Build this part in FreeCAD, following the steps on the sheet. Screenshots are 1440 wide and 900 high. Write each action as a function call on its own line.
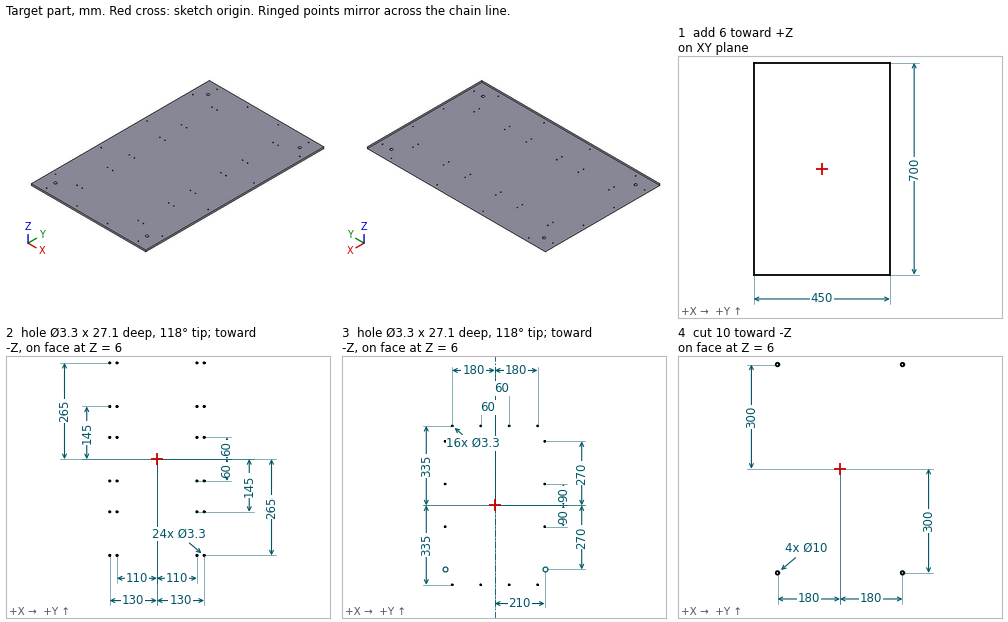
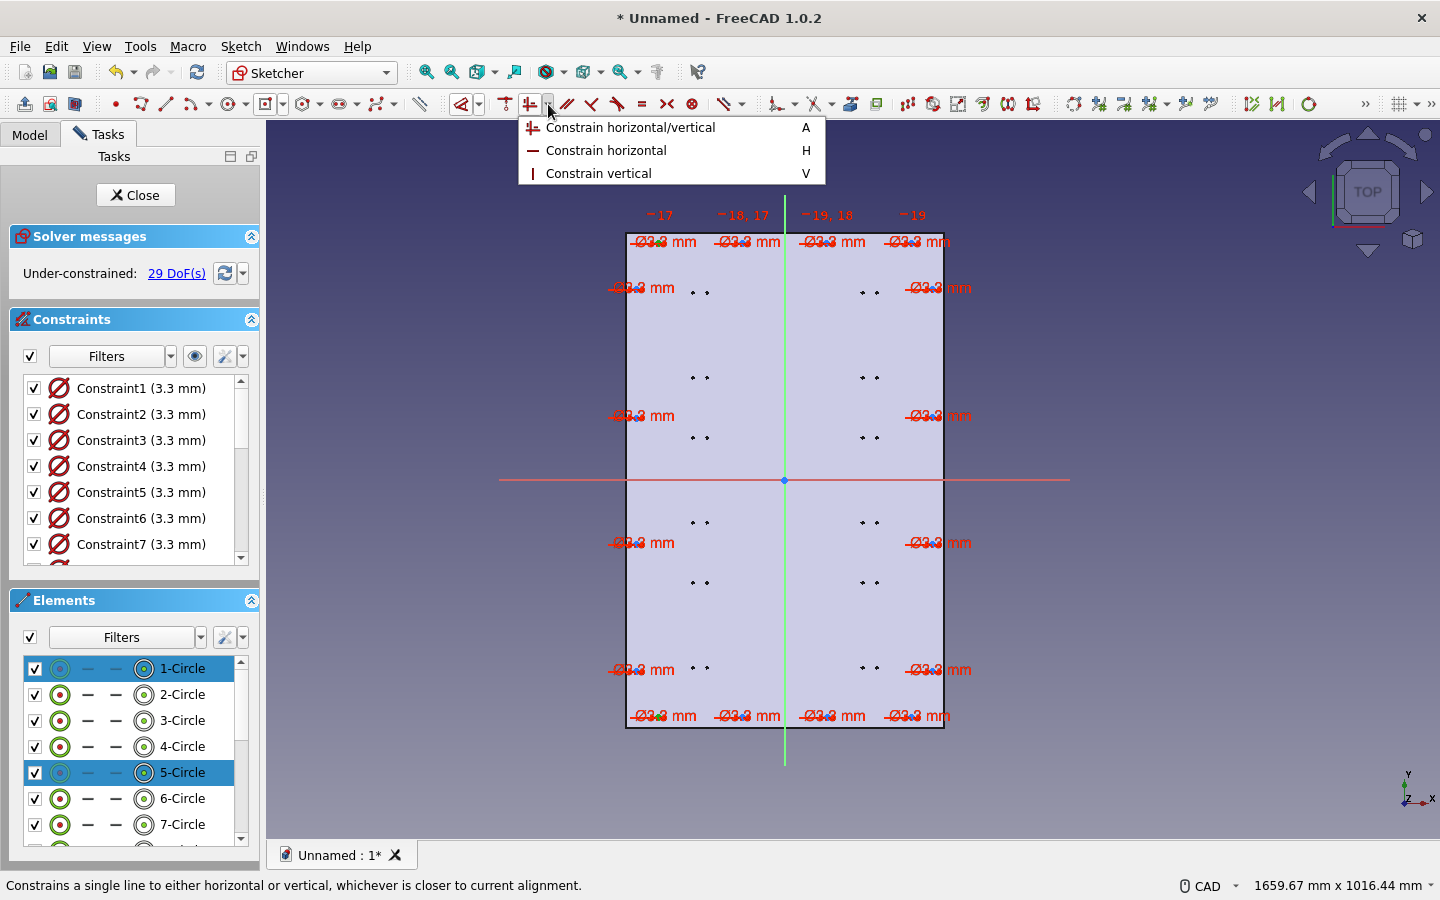
click(672, 174)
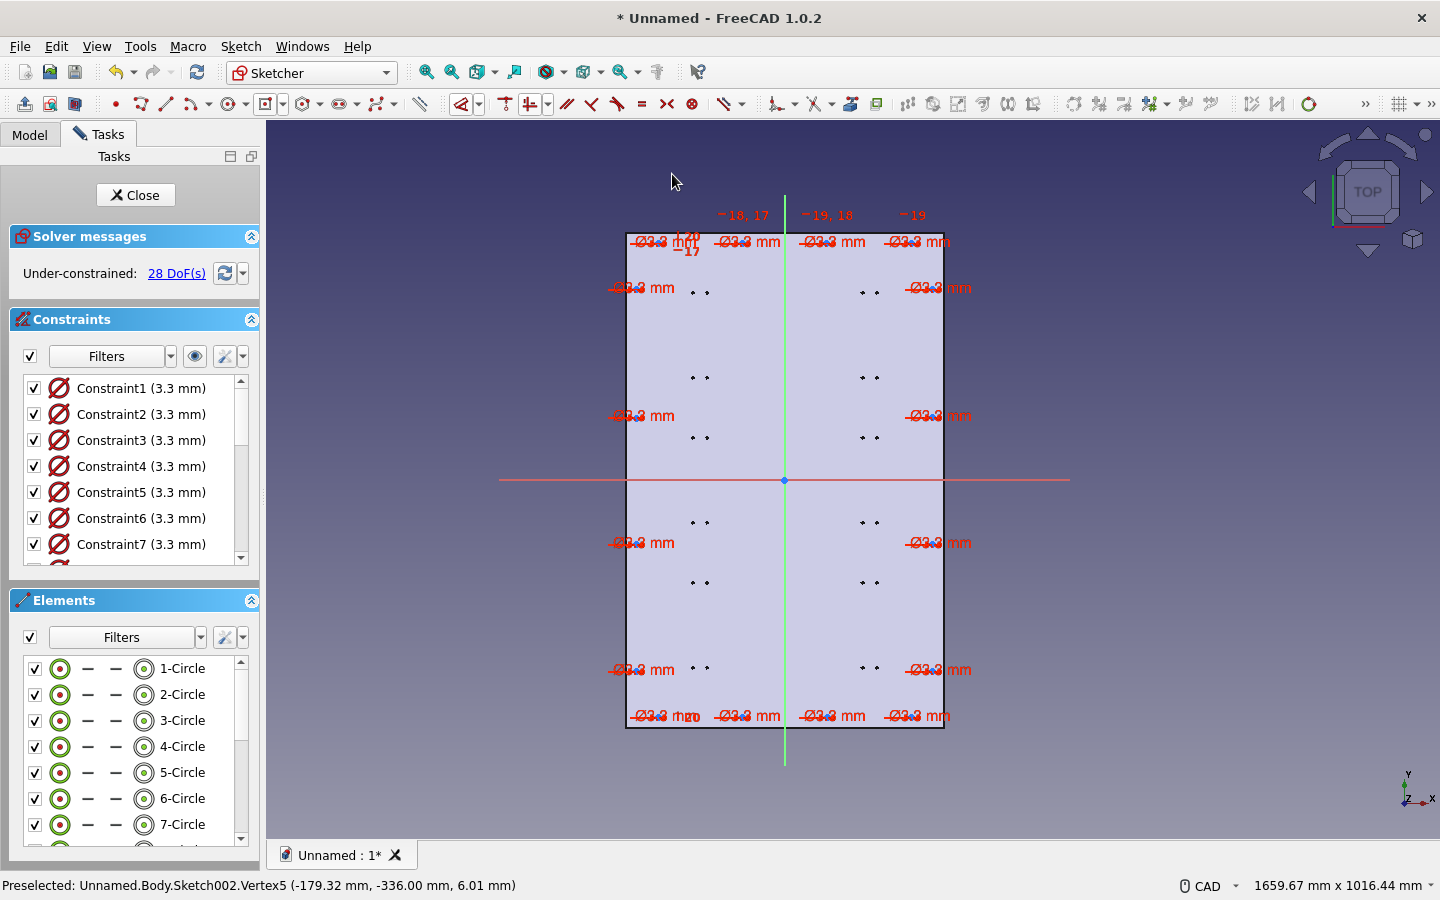
click(742, 244)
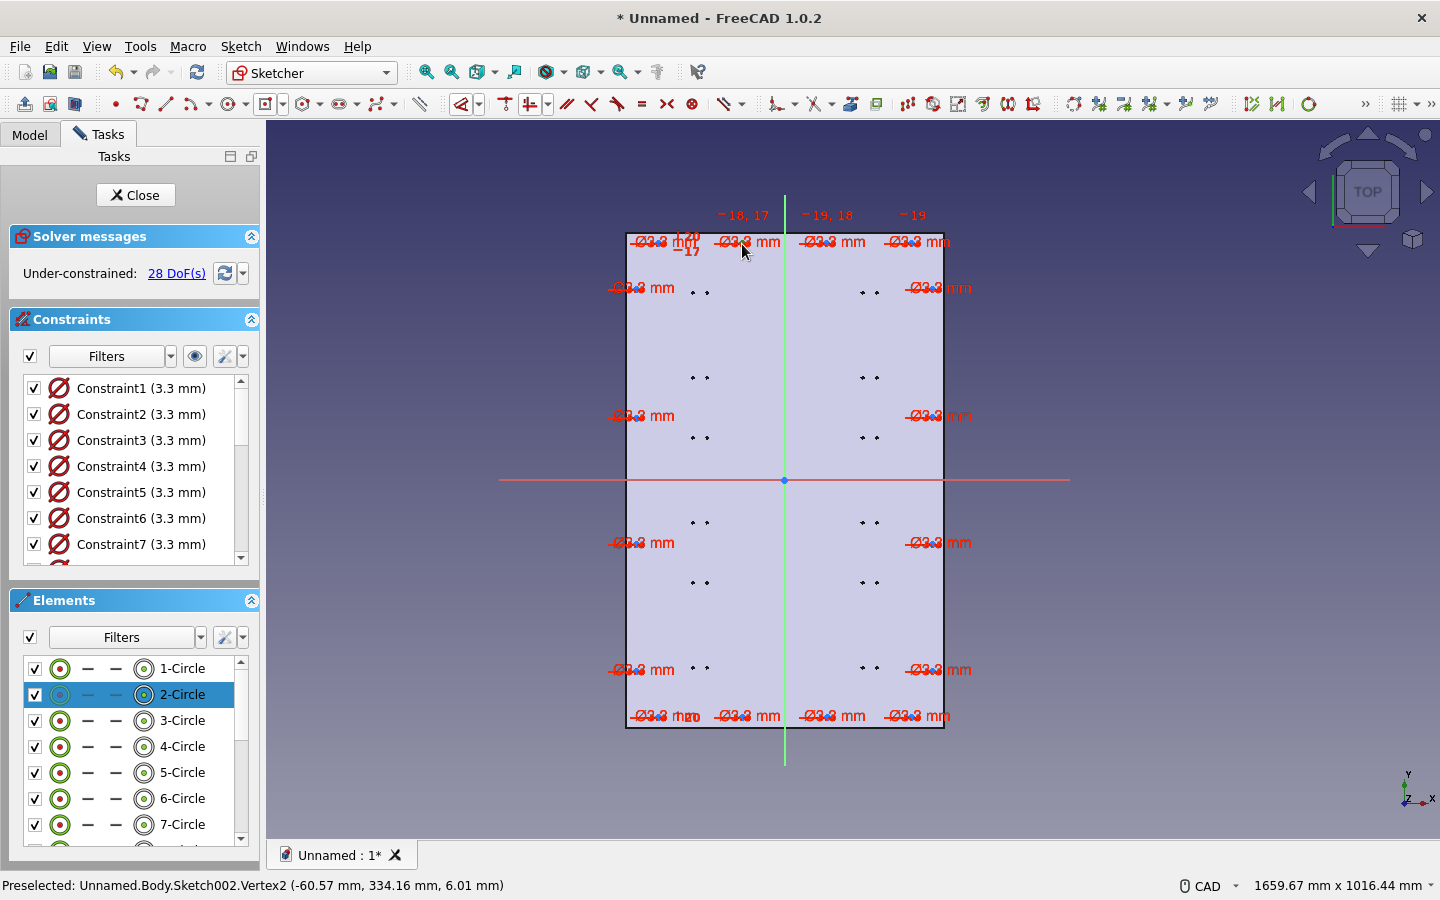
click(742, 718)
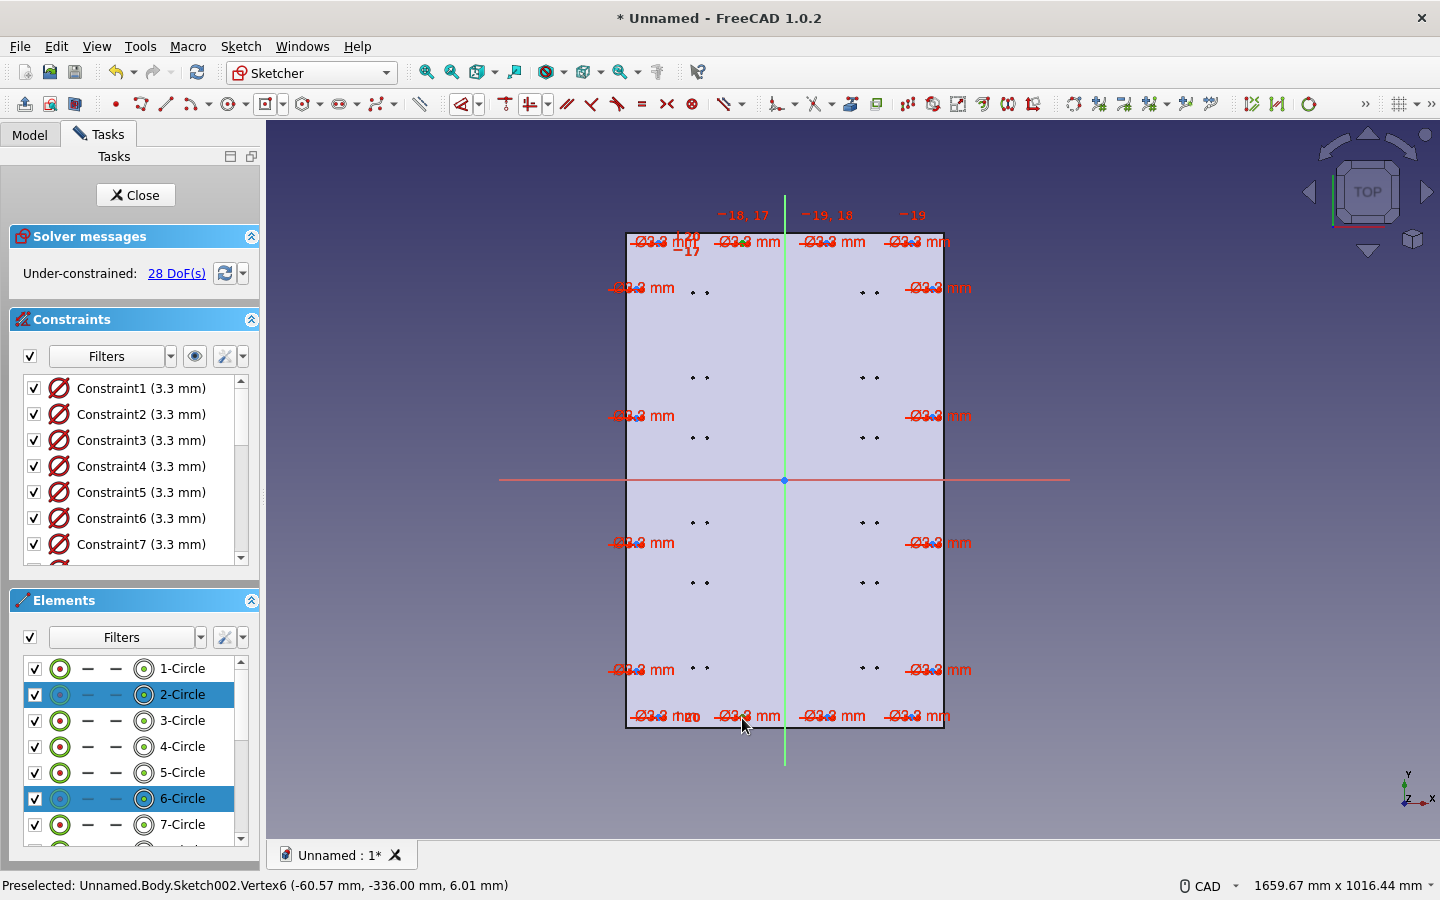
click(548, 104)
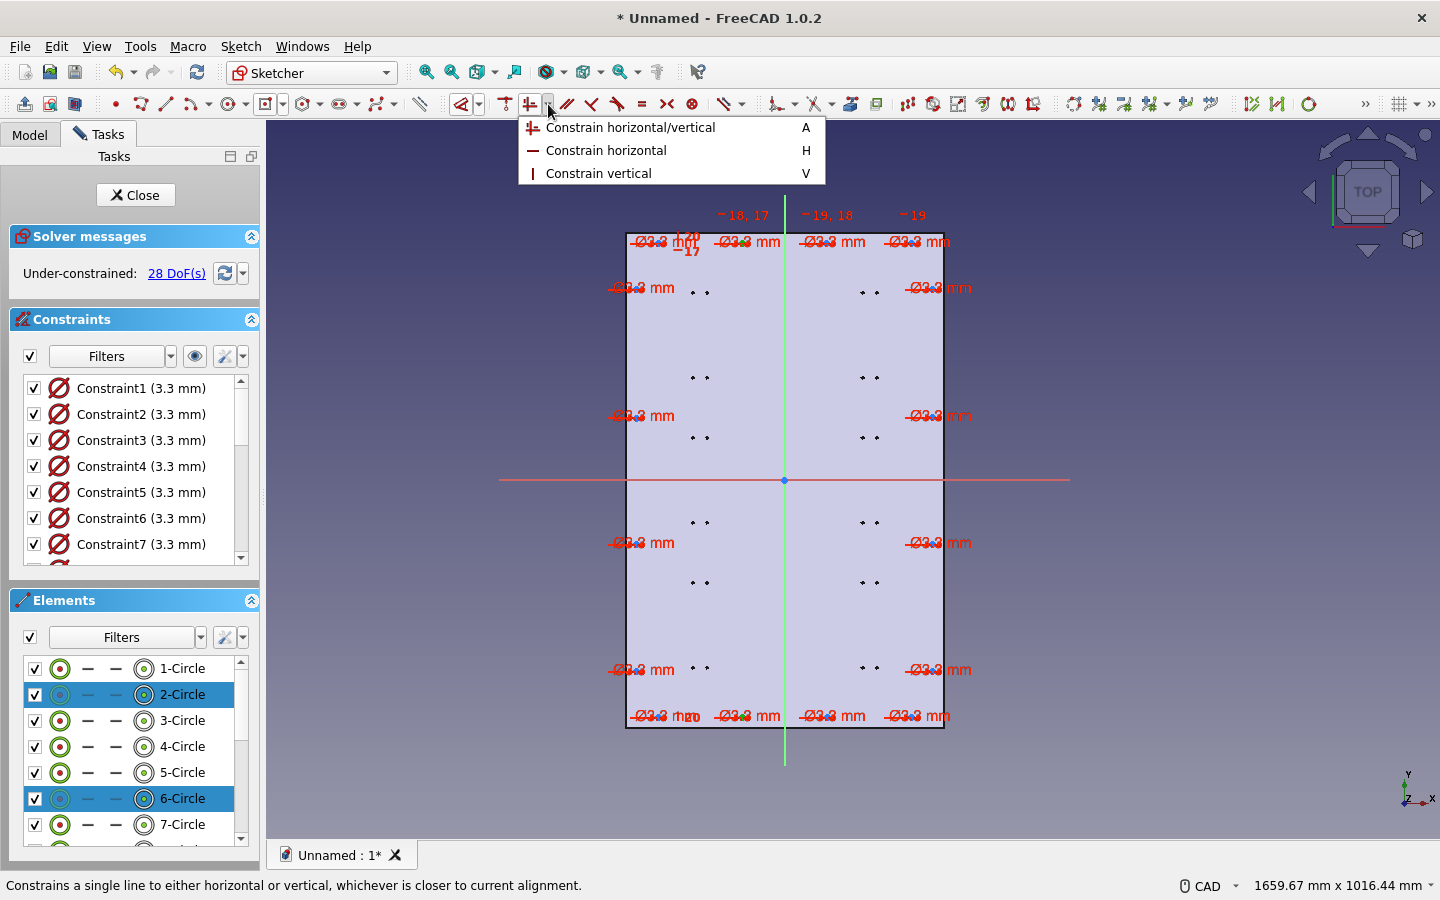
click(672, 174)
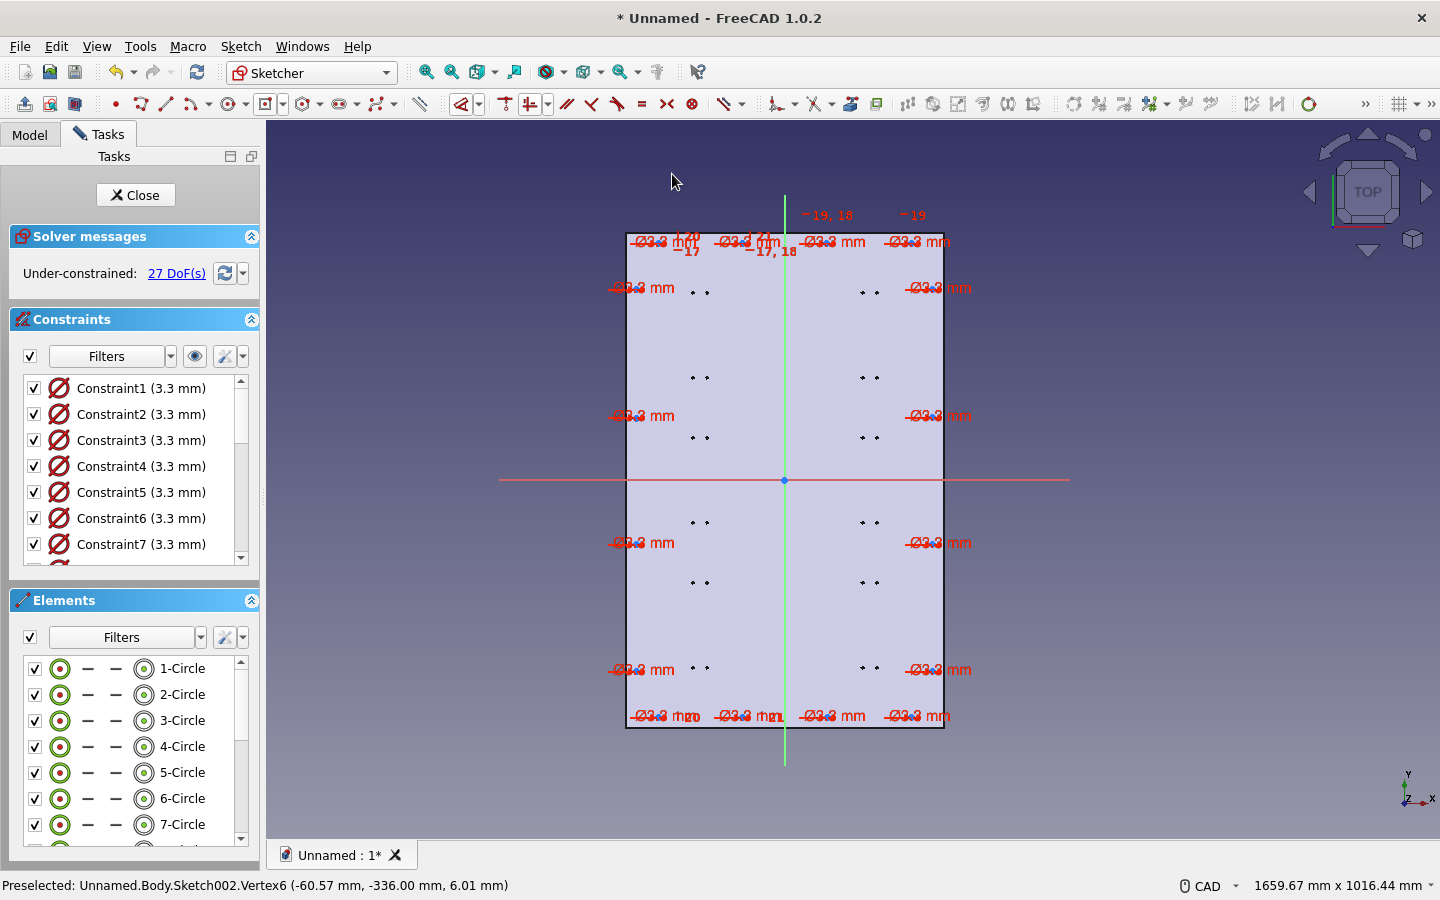
click(658, 718)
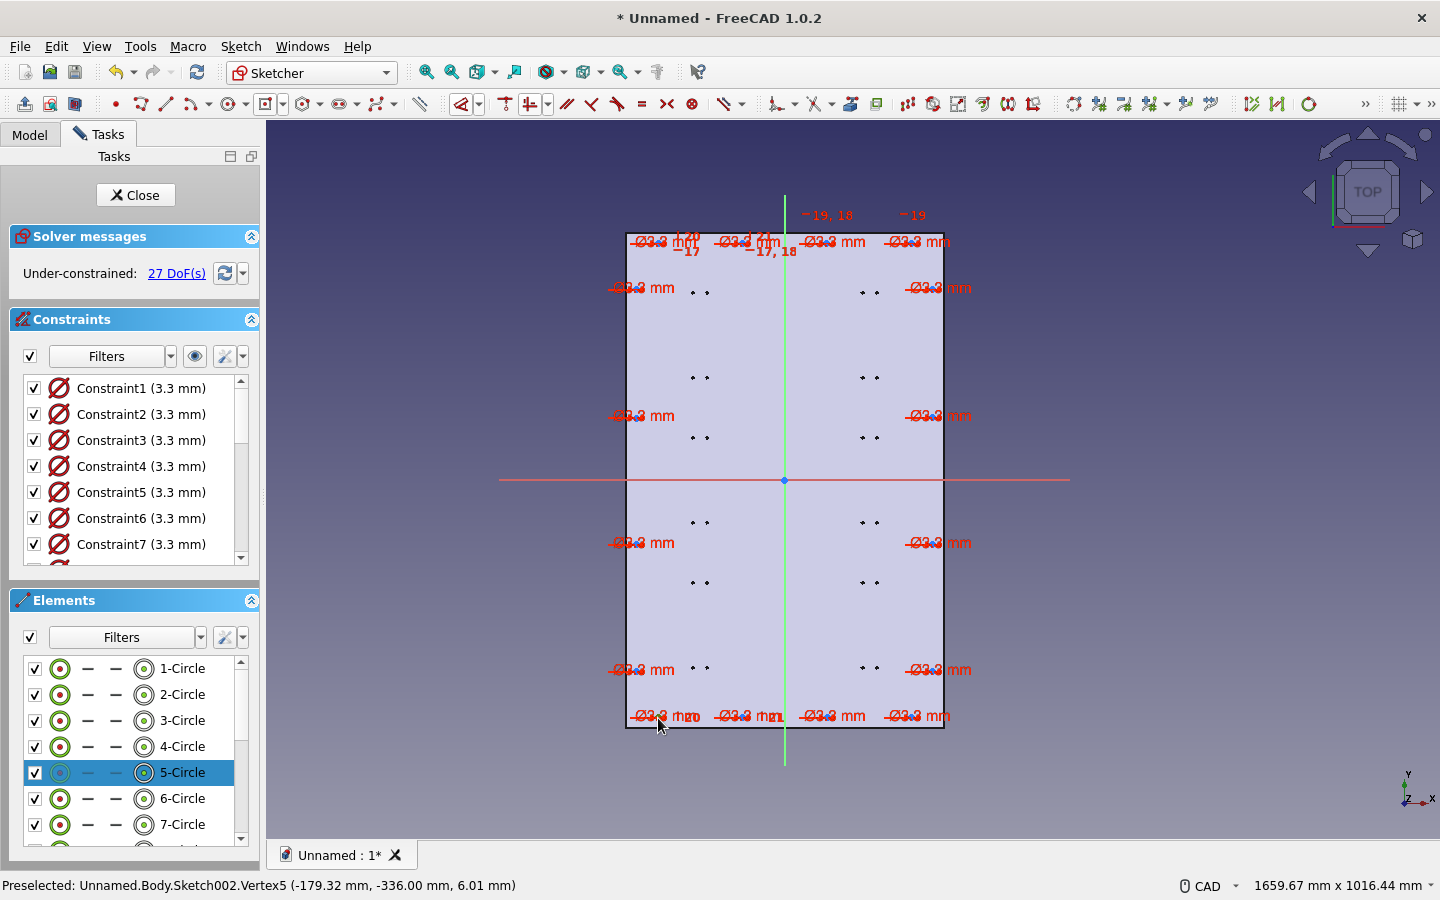
click(742, 718)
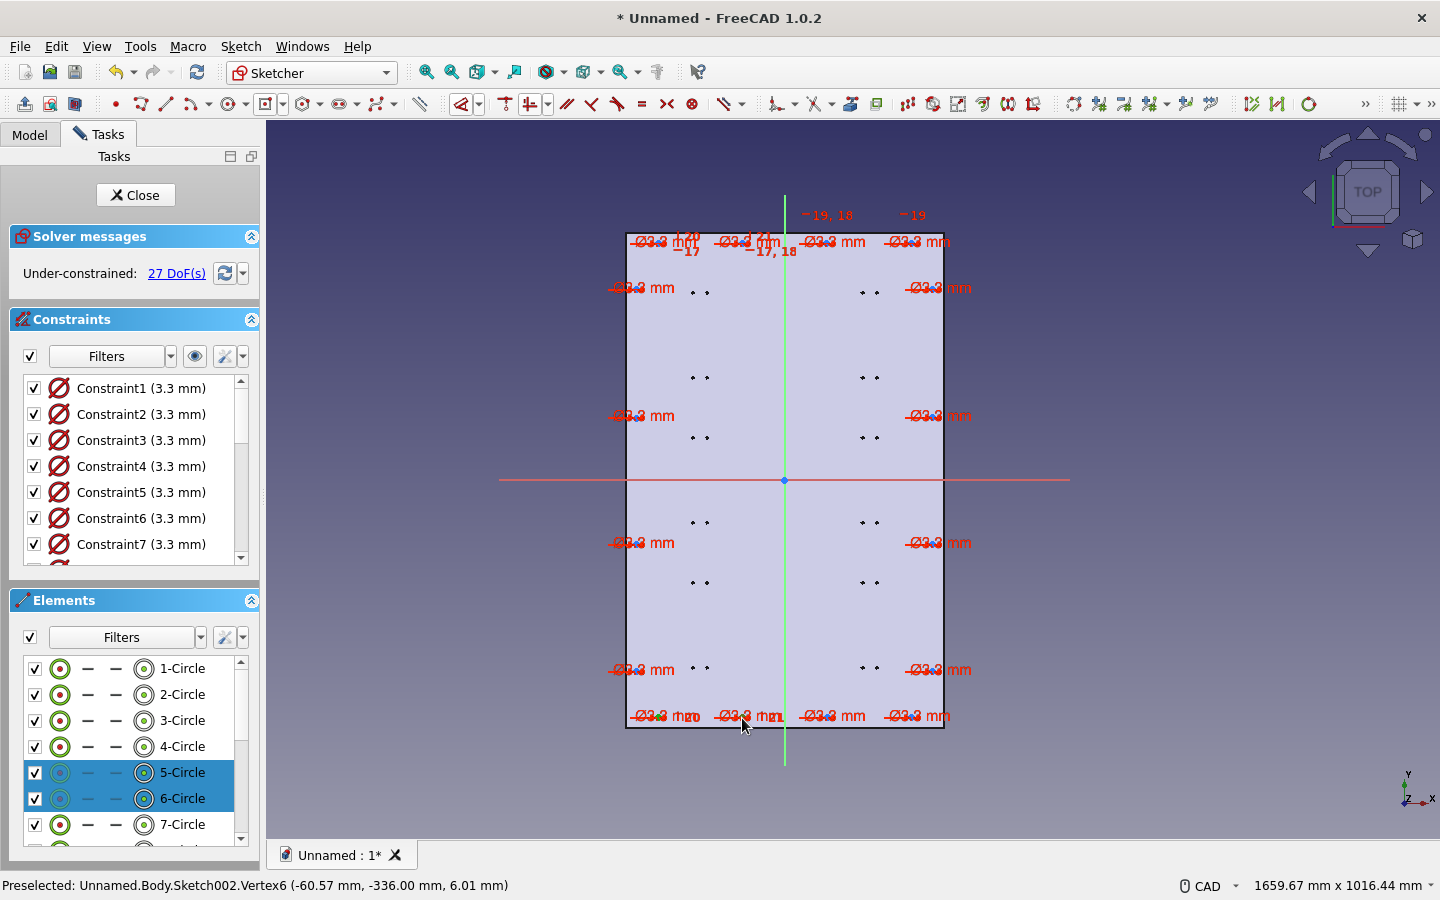
click(548, 104)